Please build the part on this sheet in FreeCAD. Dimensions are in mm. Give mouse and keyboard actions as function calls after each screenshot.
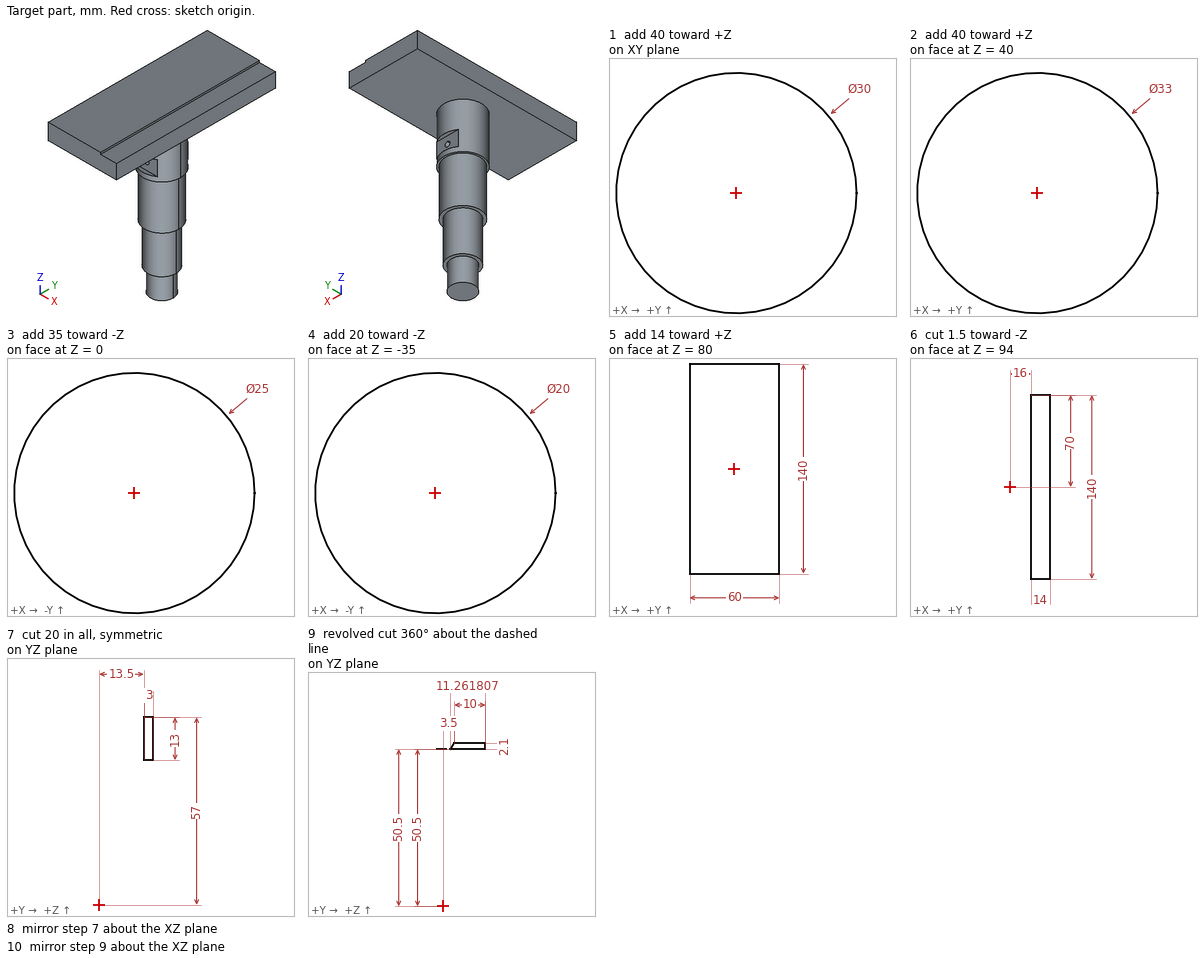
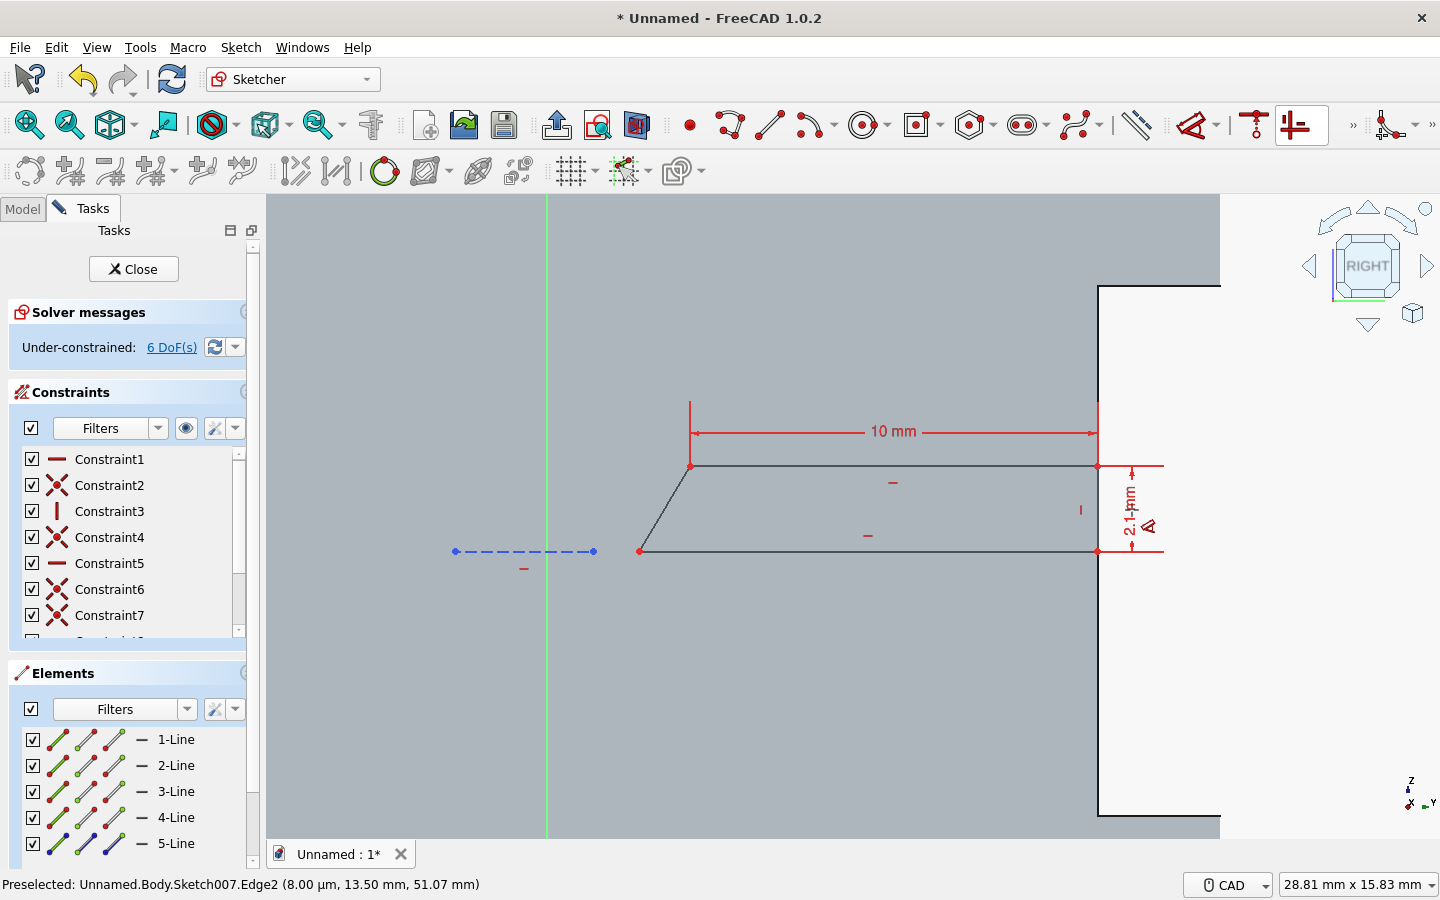
click(690, 466)
click(619, 432)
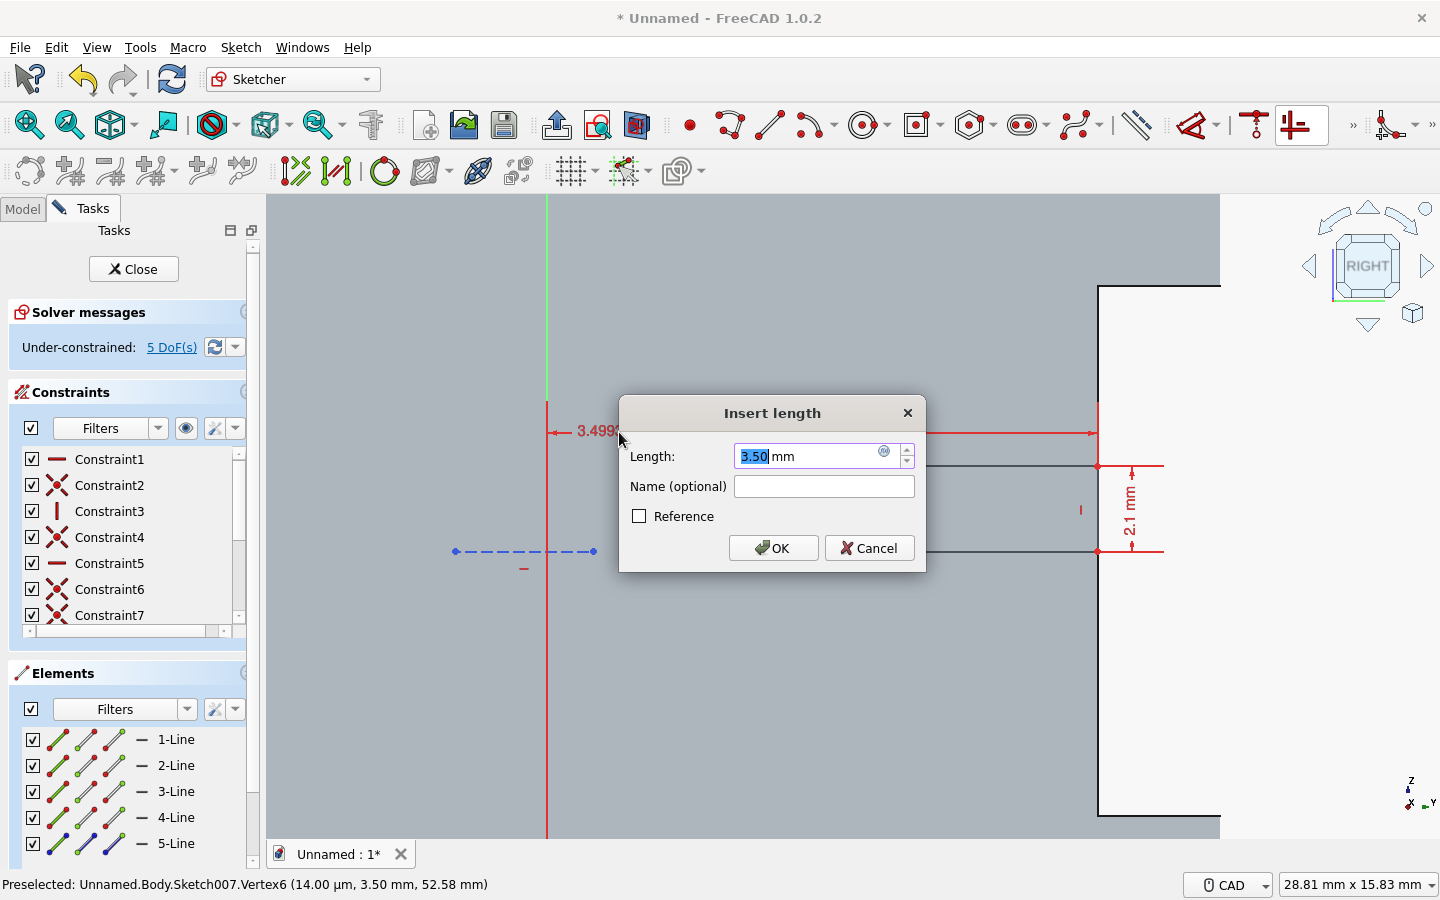
text(3.5)
key(Return)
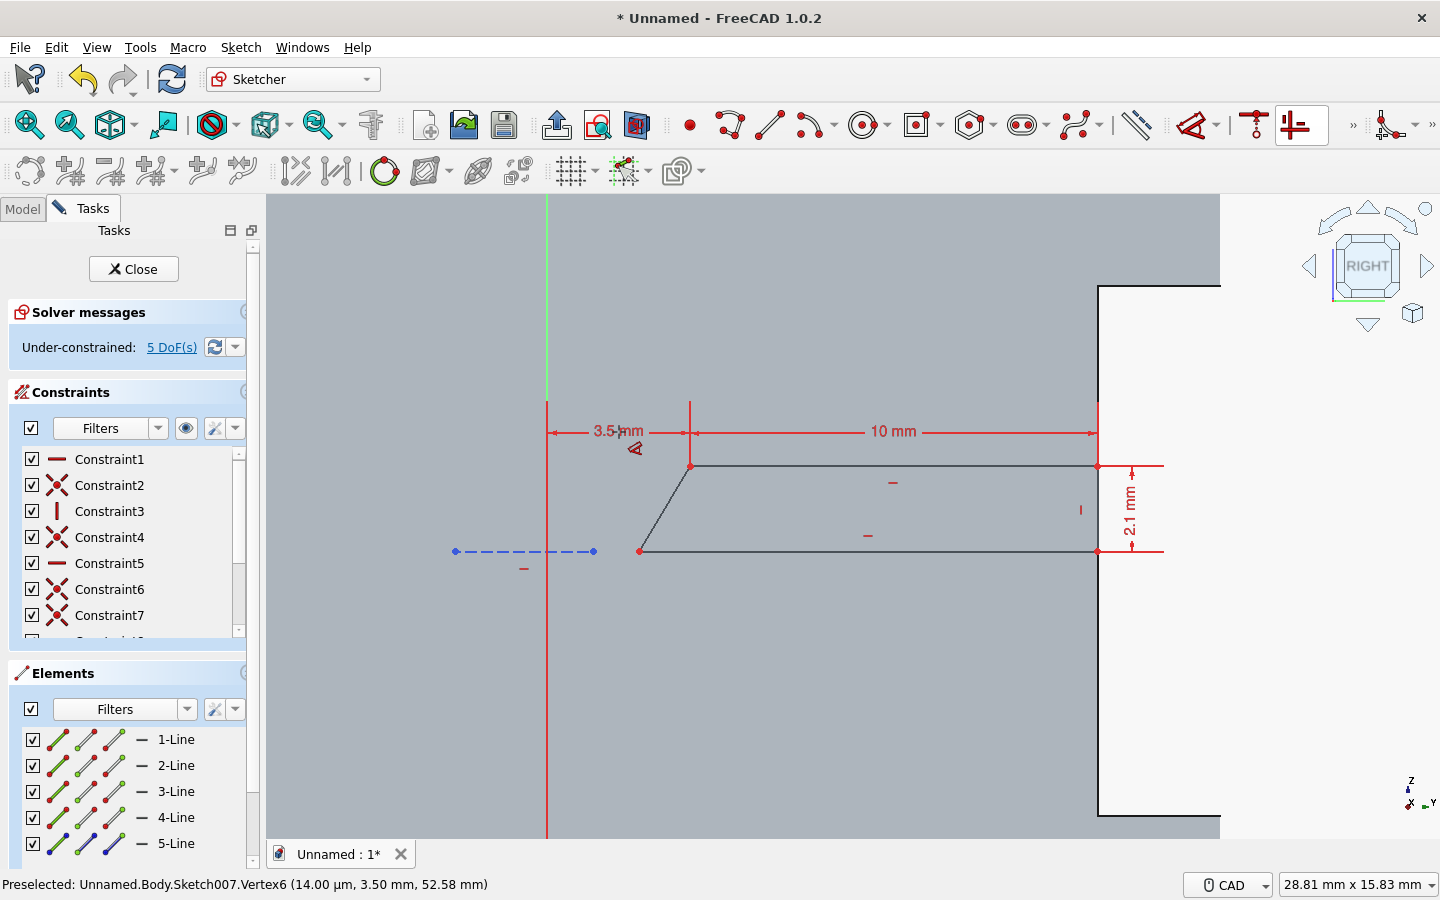
click(639, 552)
click(513, 682)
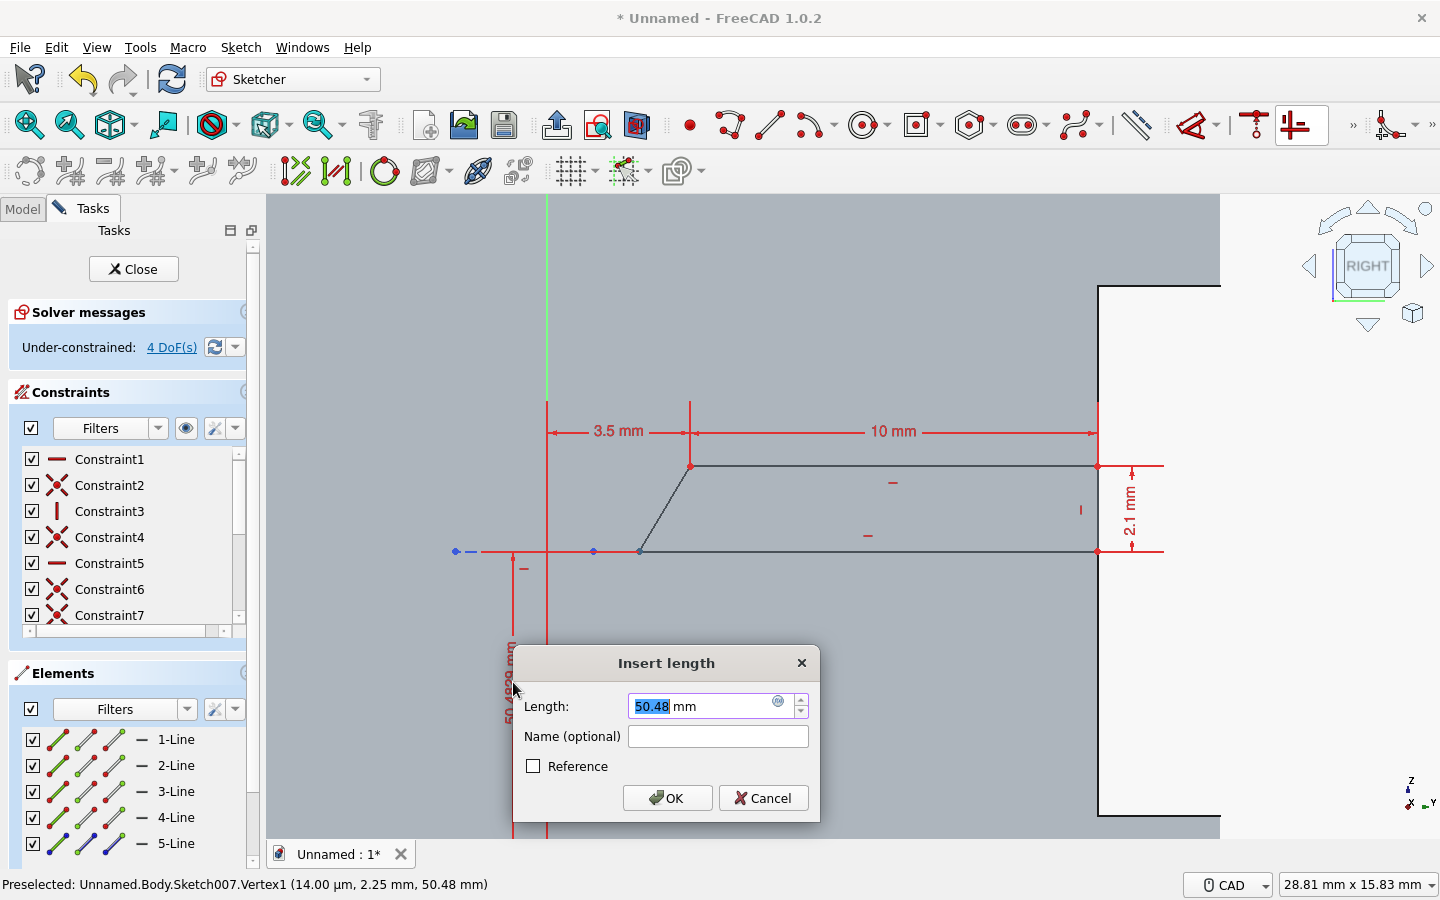
text(50.5)
key(Return)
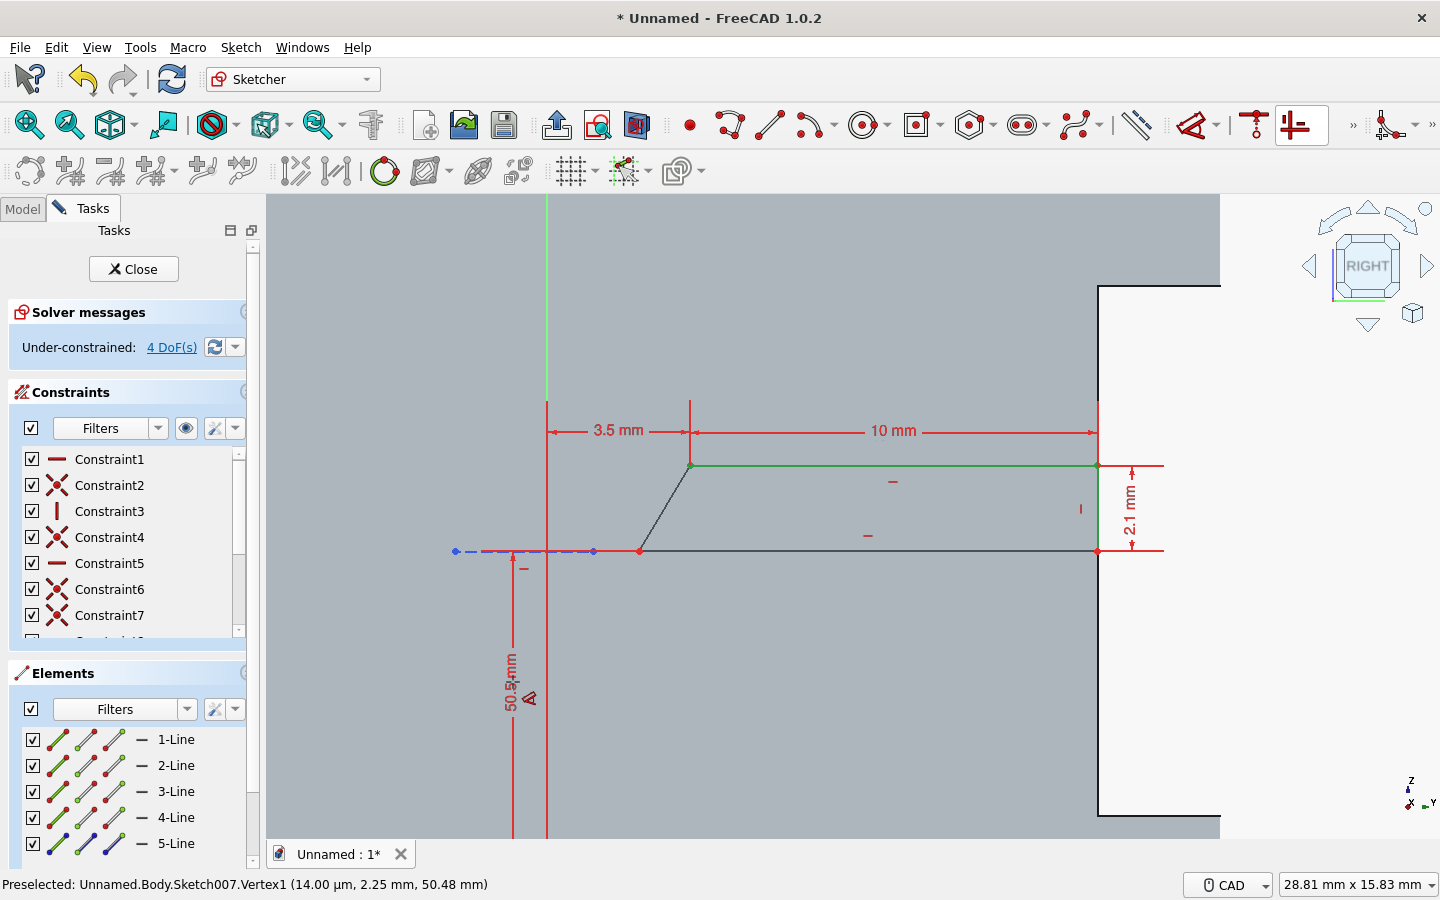
click(593, 552)
click(513, 622)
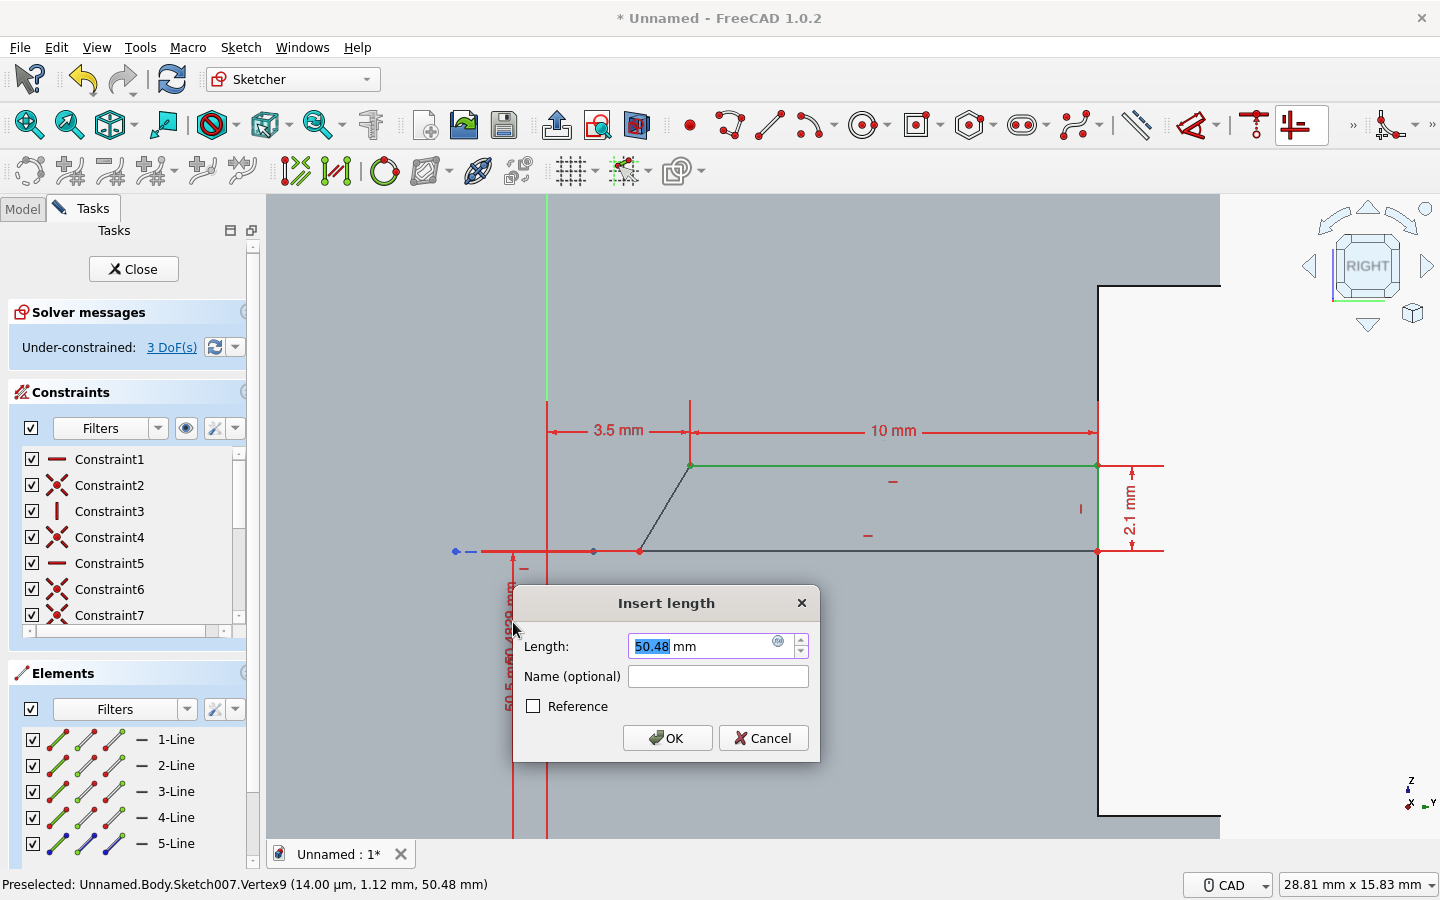
text(50.5)
key(Return)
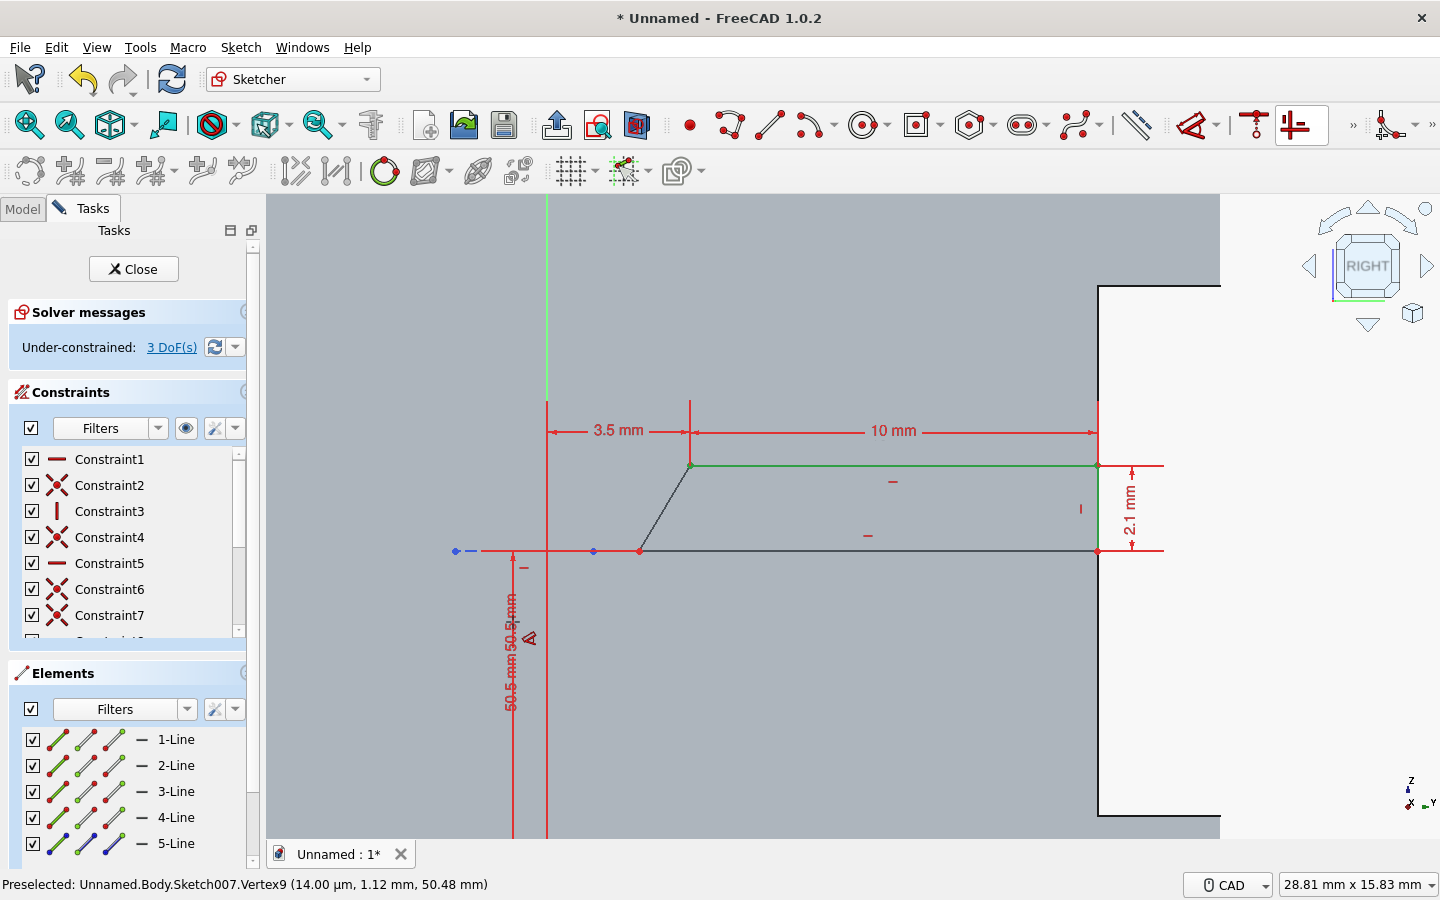
click(777, 551)
click(868, 585)